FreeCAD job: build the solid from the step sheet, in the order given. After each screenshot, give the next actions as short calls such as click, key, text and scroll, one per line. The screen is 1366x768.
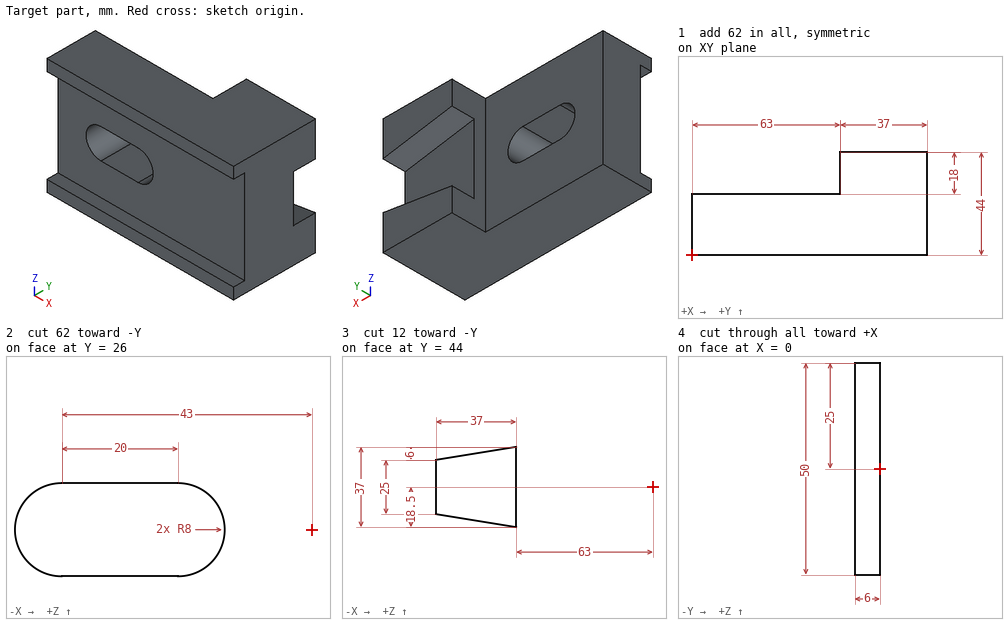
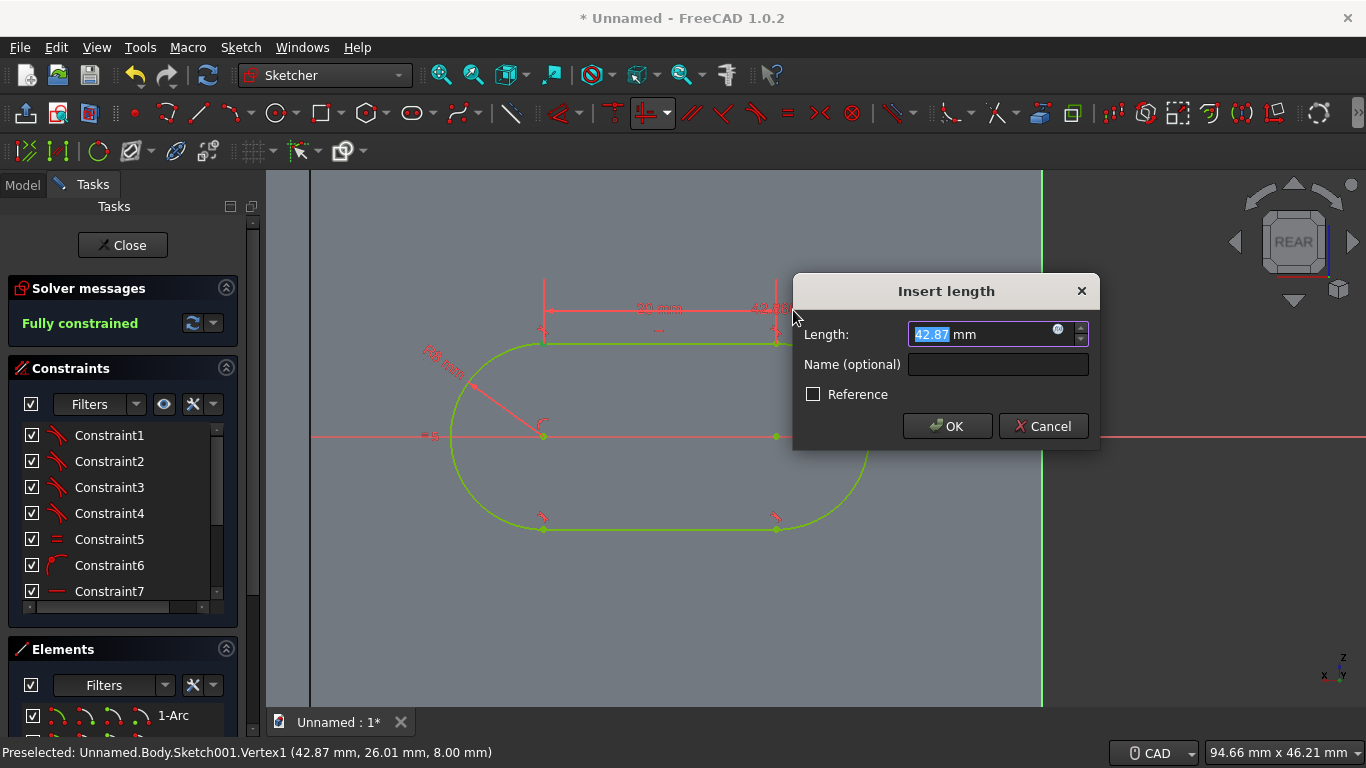
text(43)
key(Return)
key(Escape)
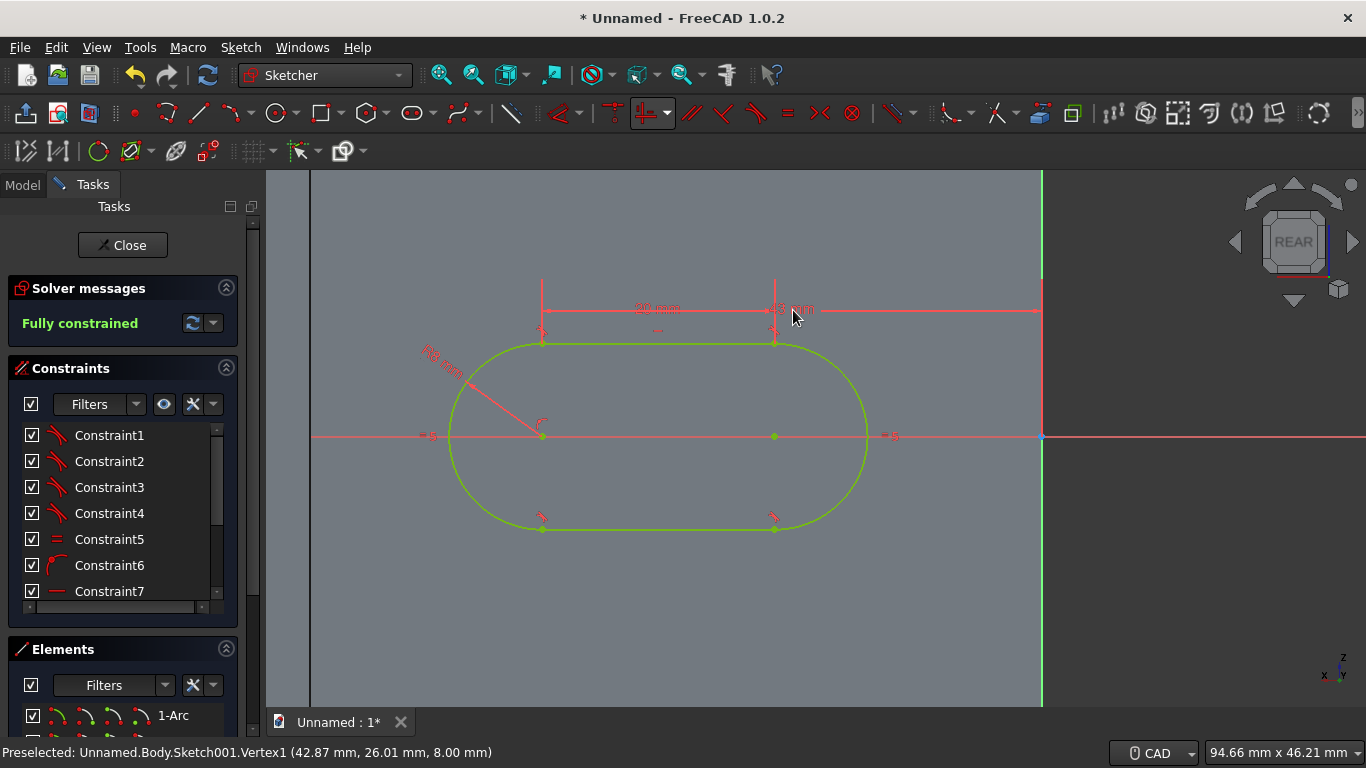
click(123, 245)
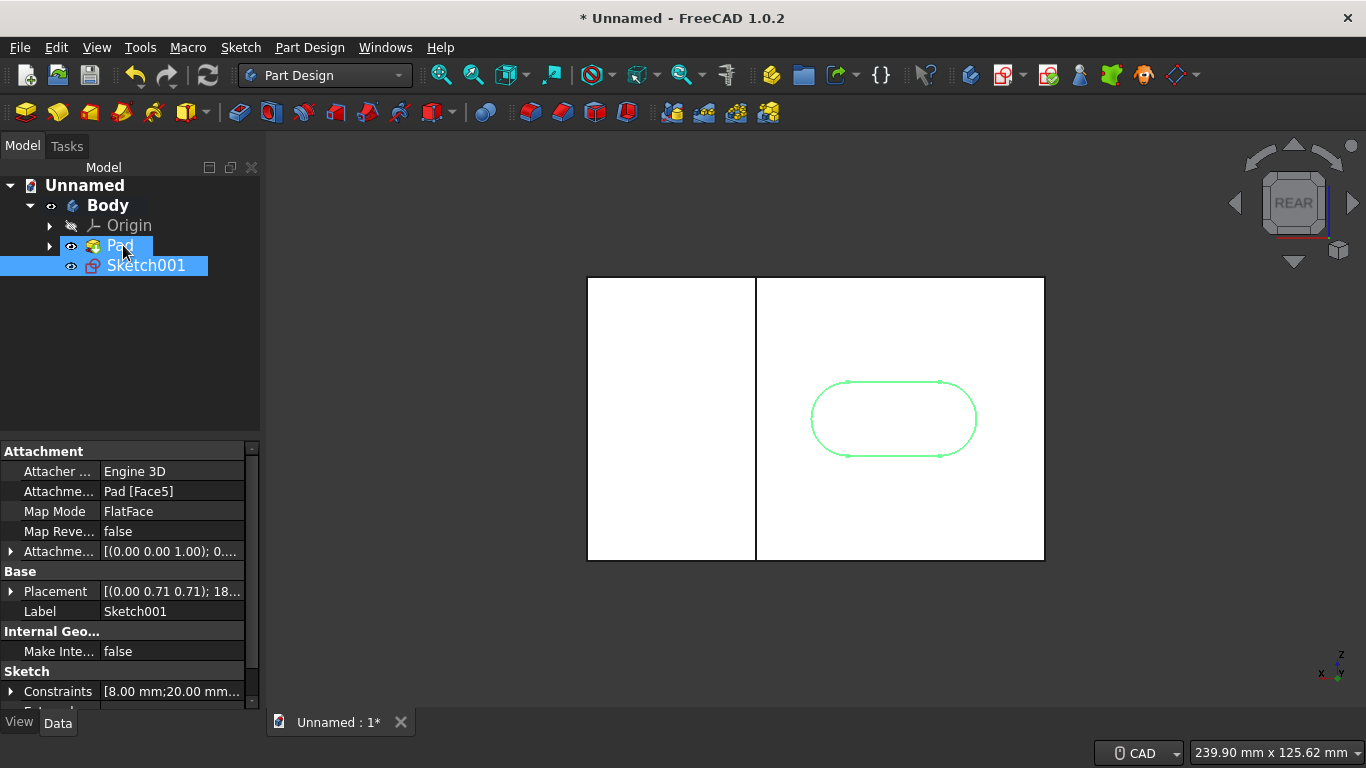
click(240, 112)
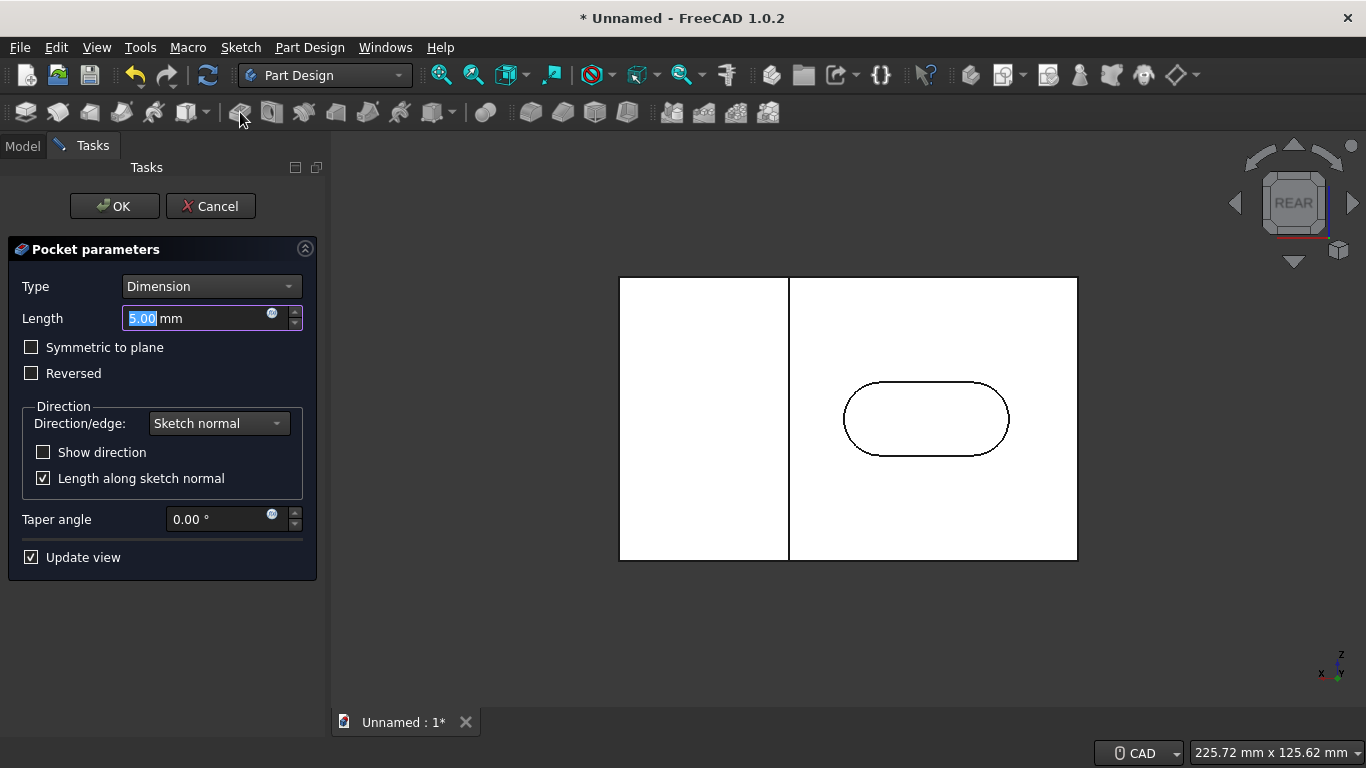
text(62)
key(Tab)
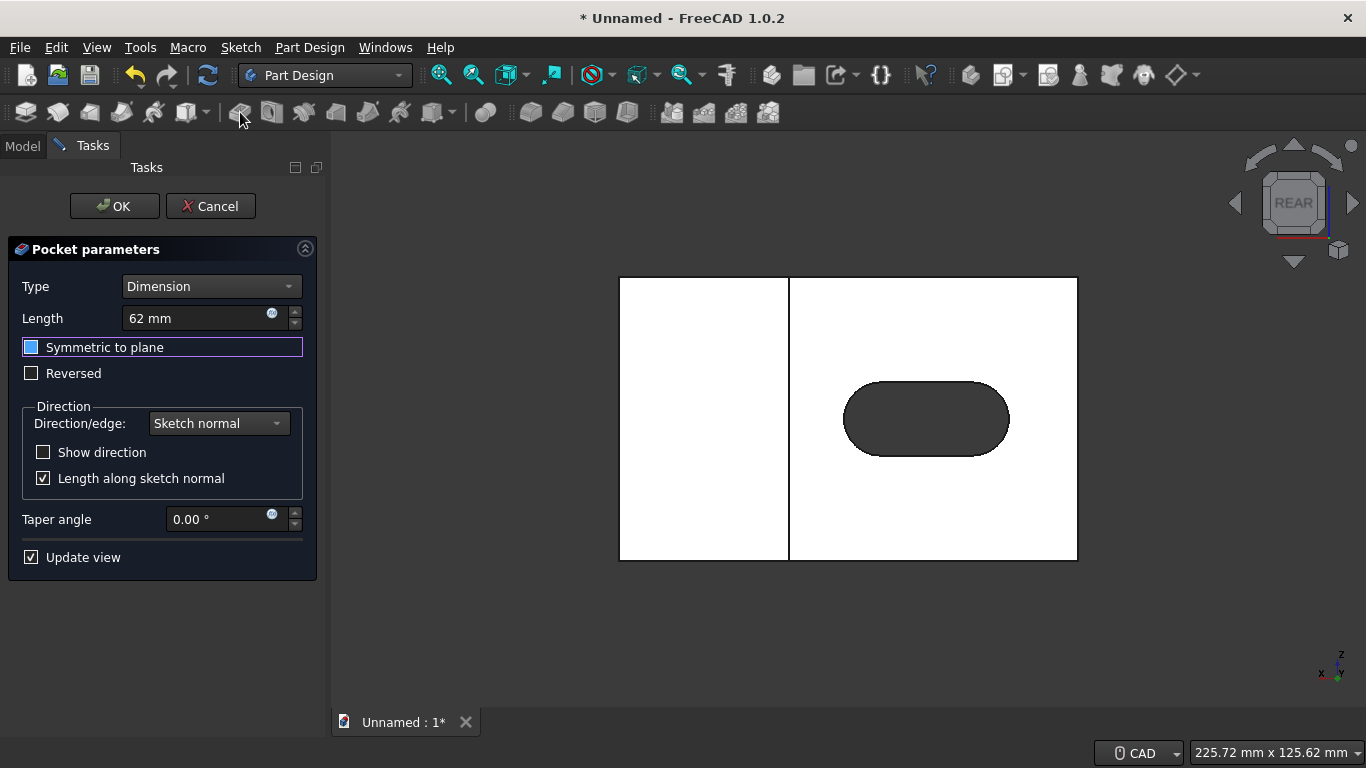
click(115, 206)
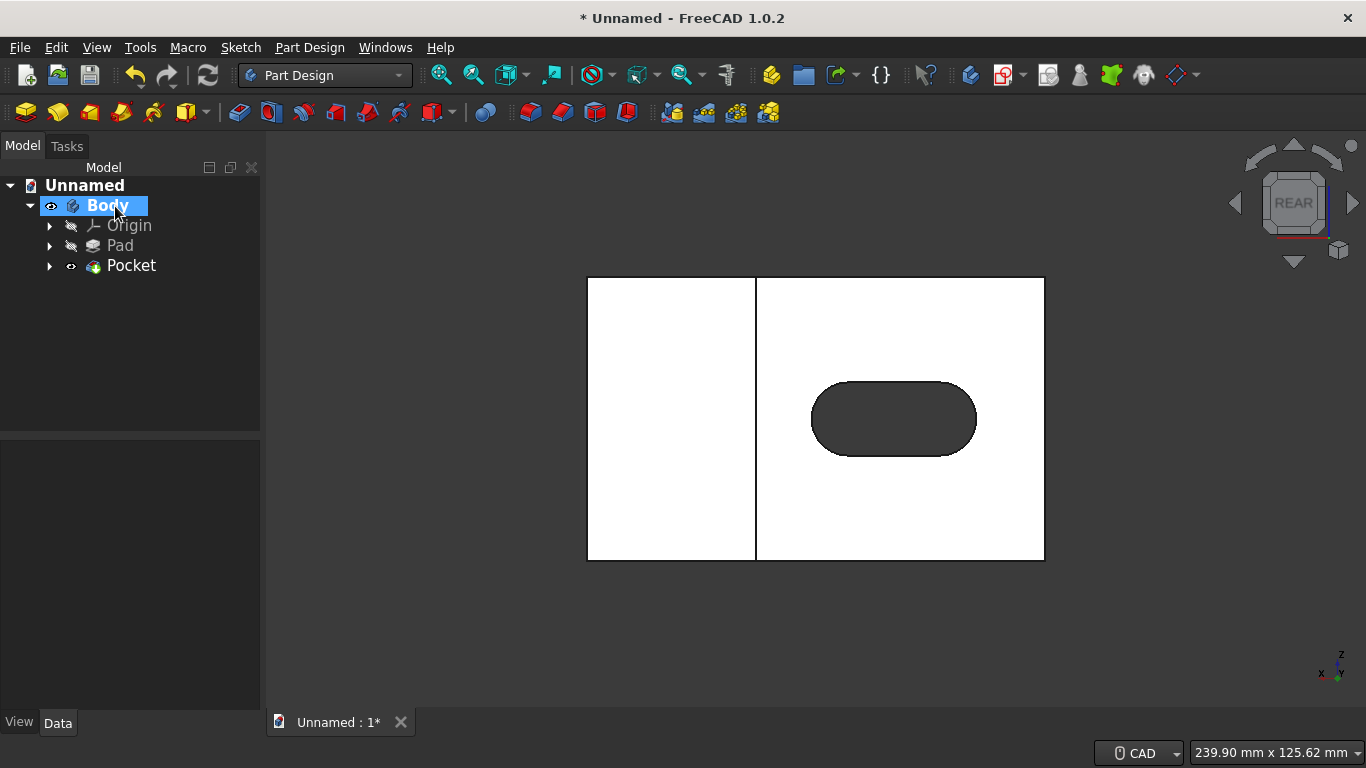
click(672, 377)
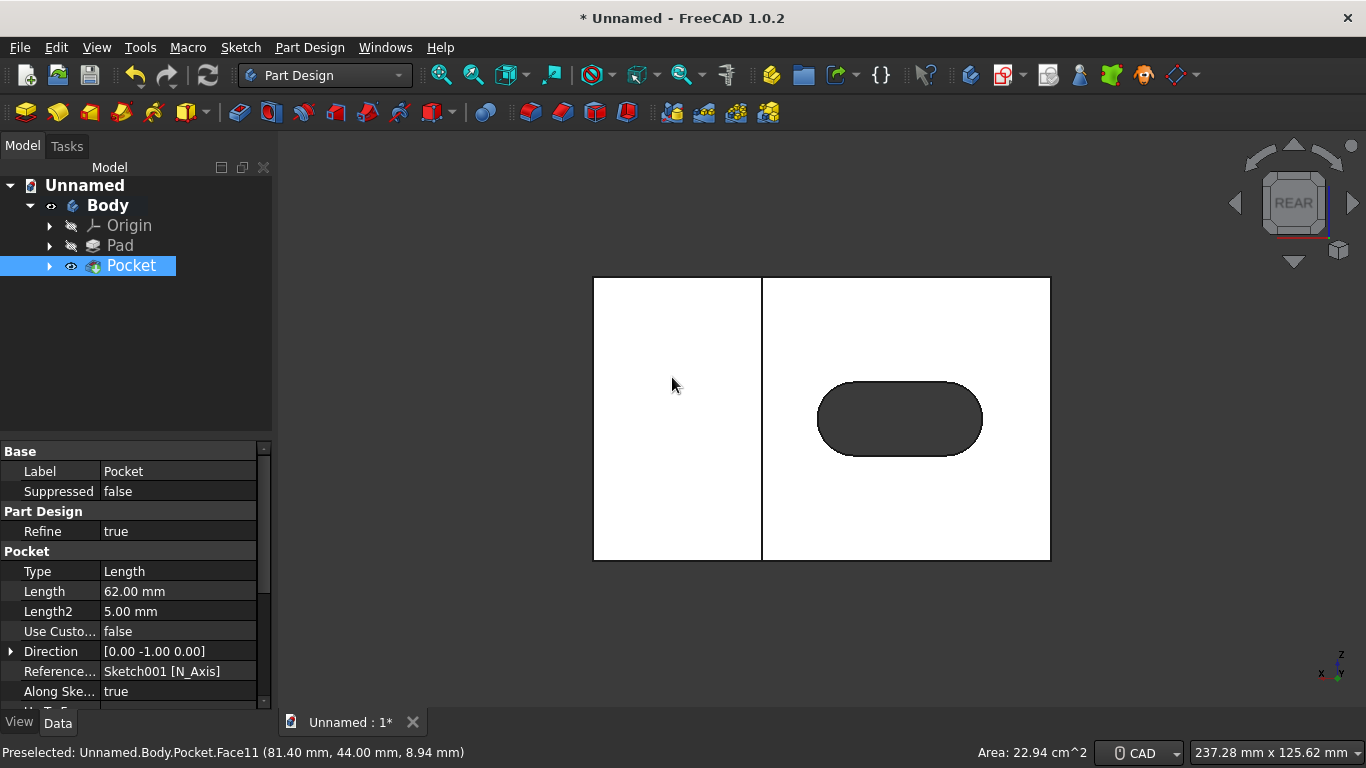
click(1004, 76)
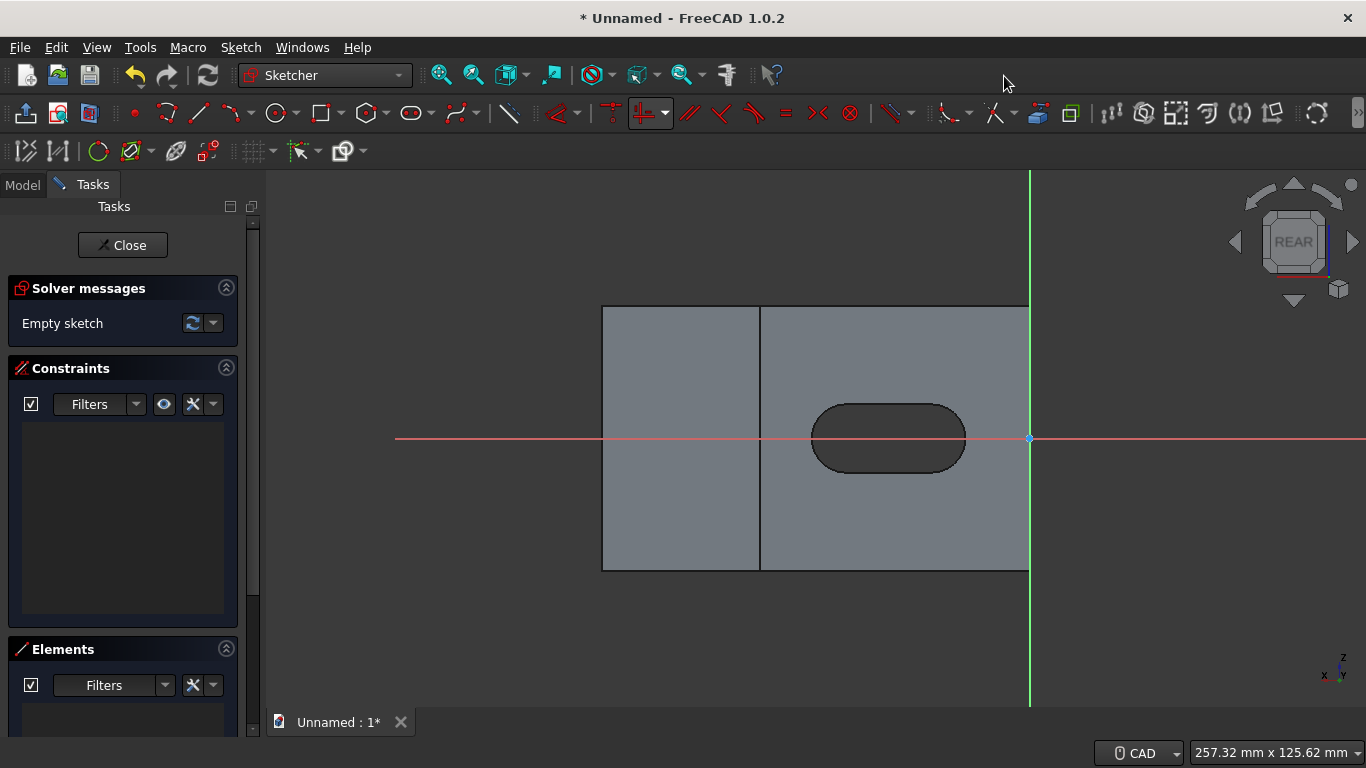
scroll(627, 439, up, 4)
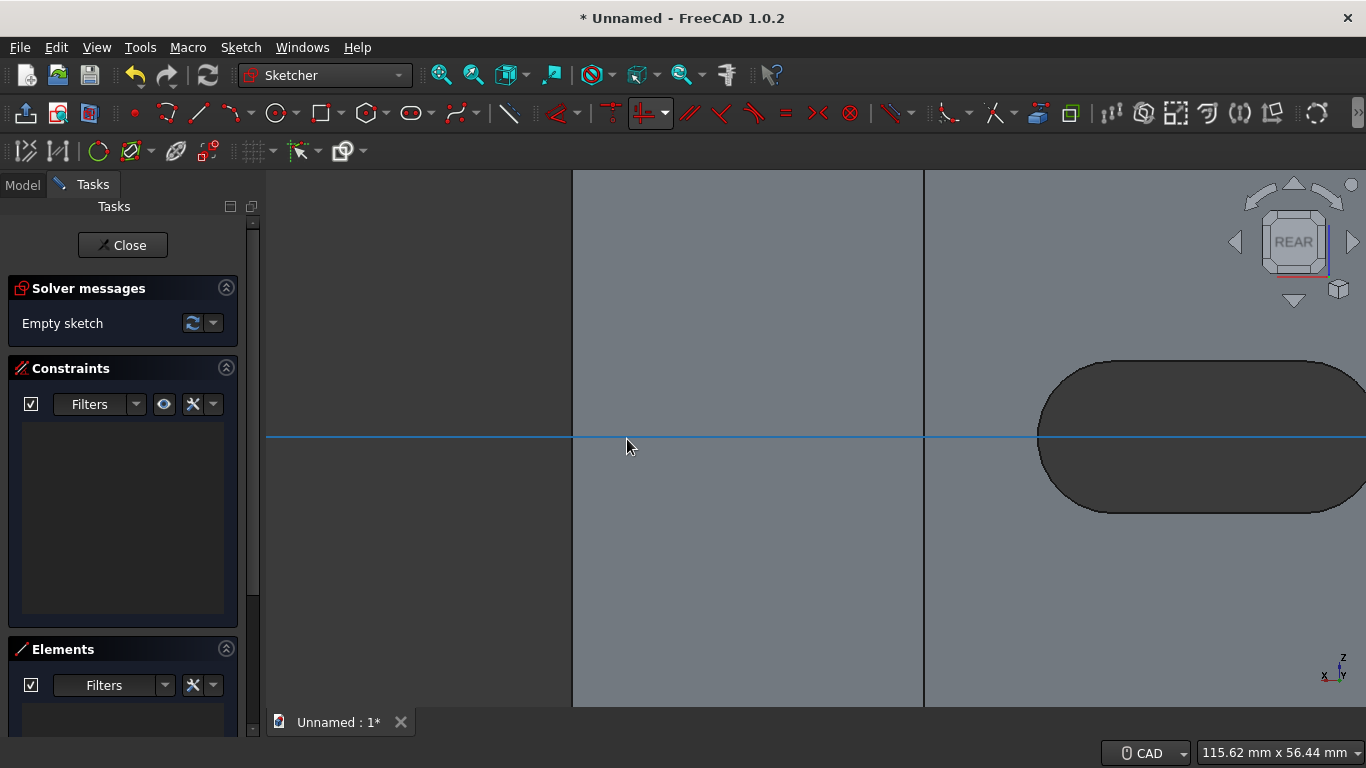
click(168, 114)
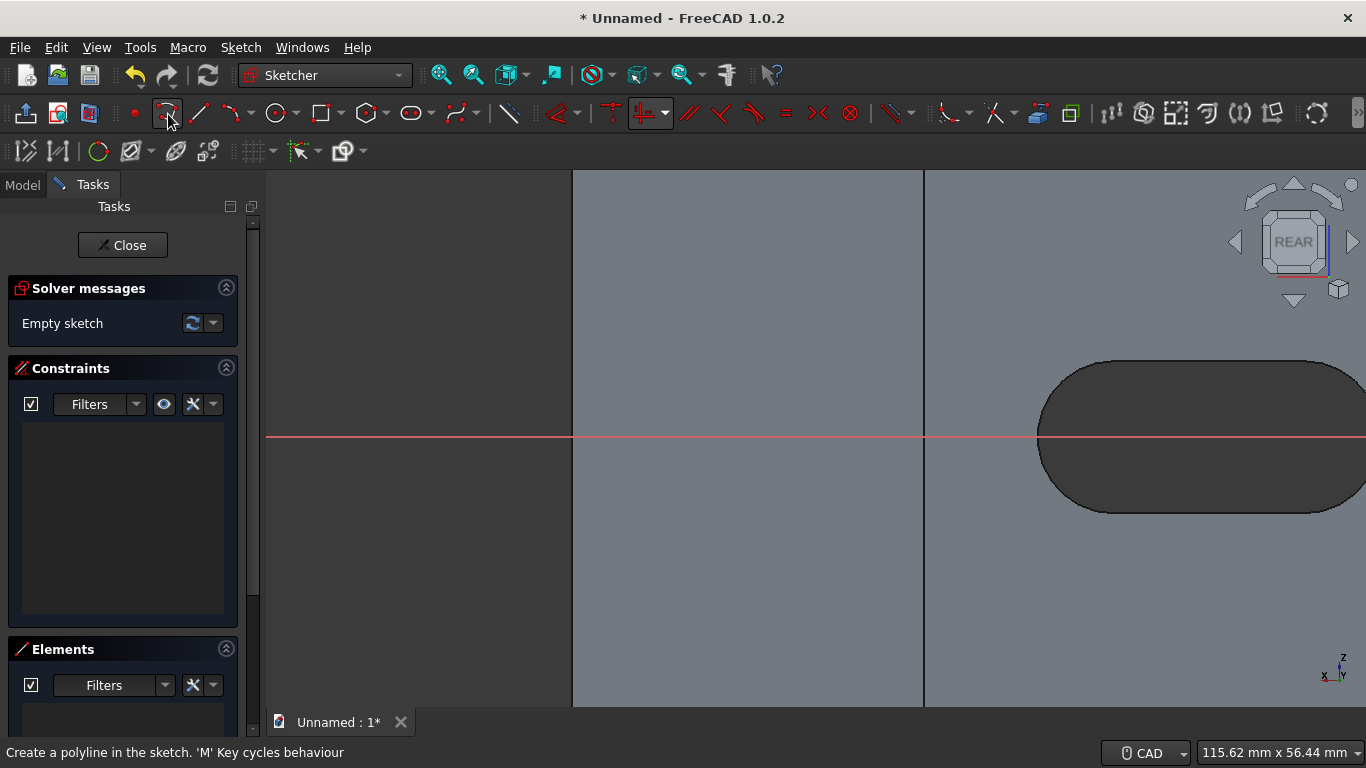
click(924, 613)
click(924, 261)
click(572, 318)
click(572, 556)
click(924, 614)
key(Escape)
key(Escape)